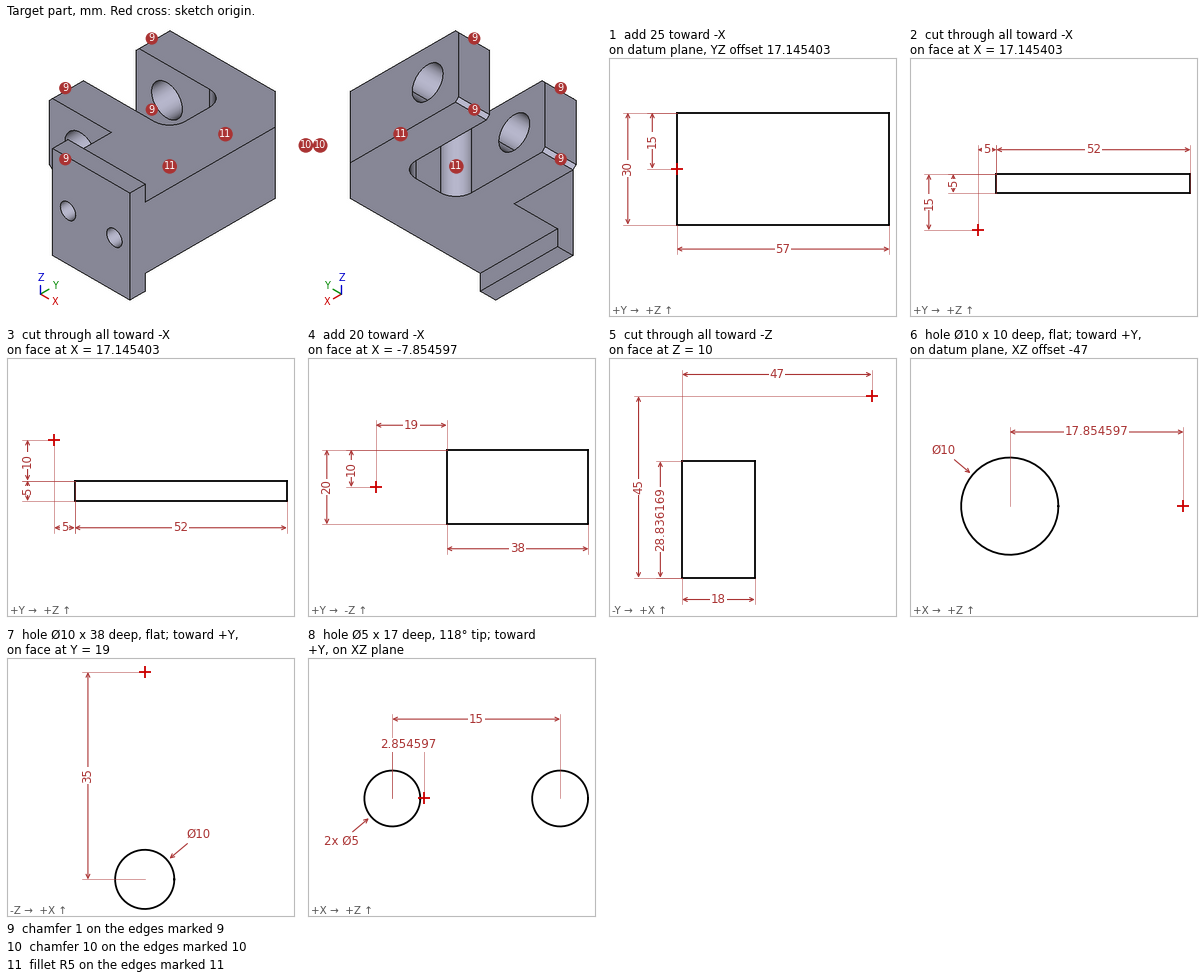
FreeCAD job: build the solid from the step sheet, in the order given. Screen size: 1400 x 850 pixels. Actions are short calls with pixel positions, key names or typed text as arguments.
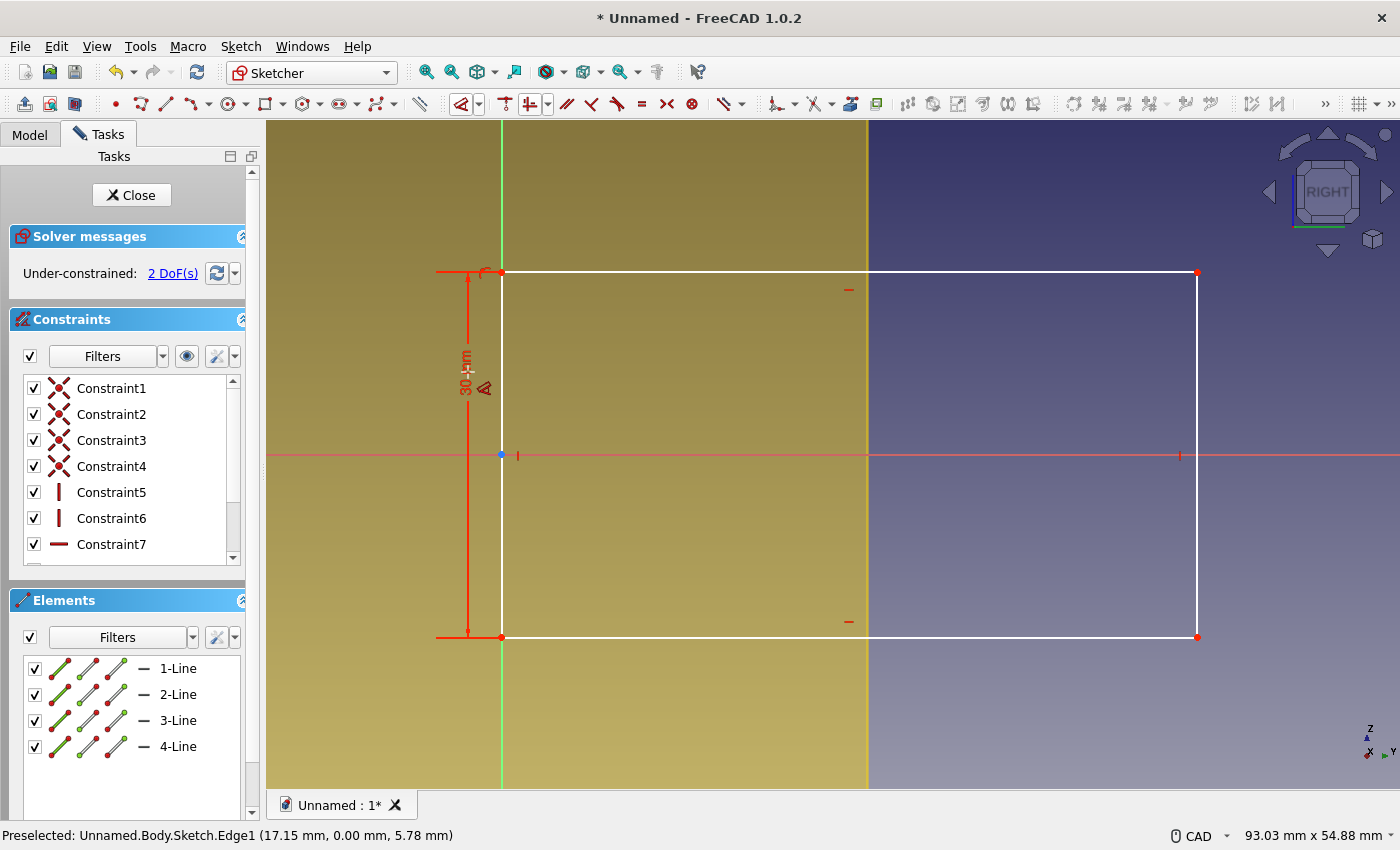
click(710, 638)
click(849, 672)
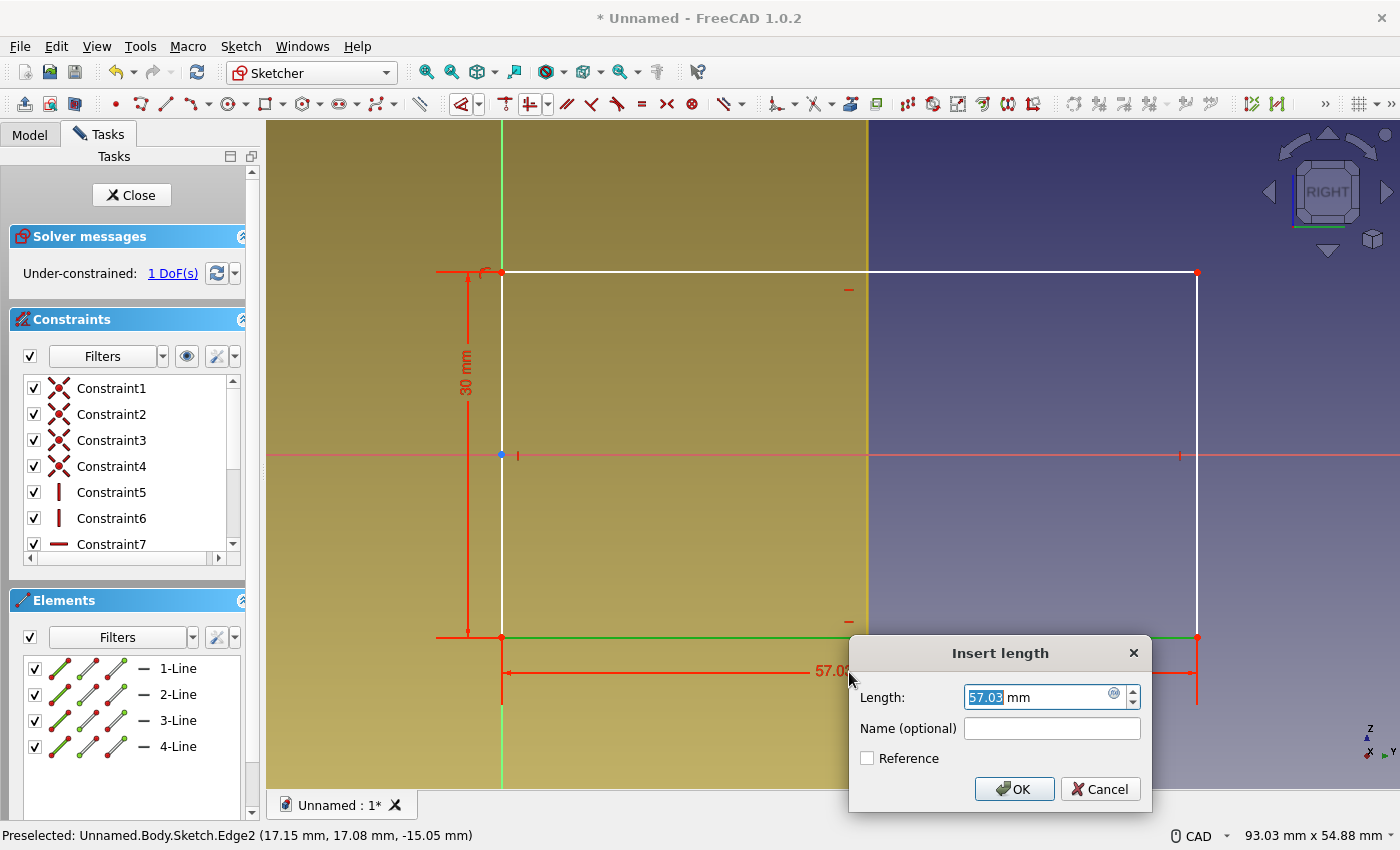
text(57)
key(Return)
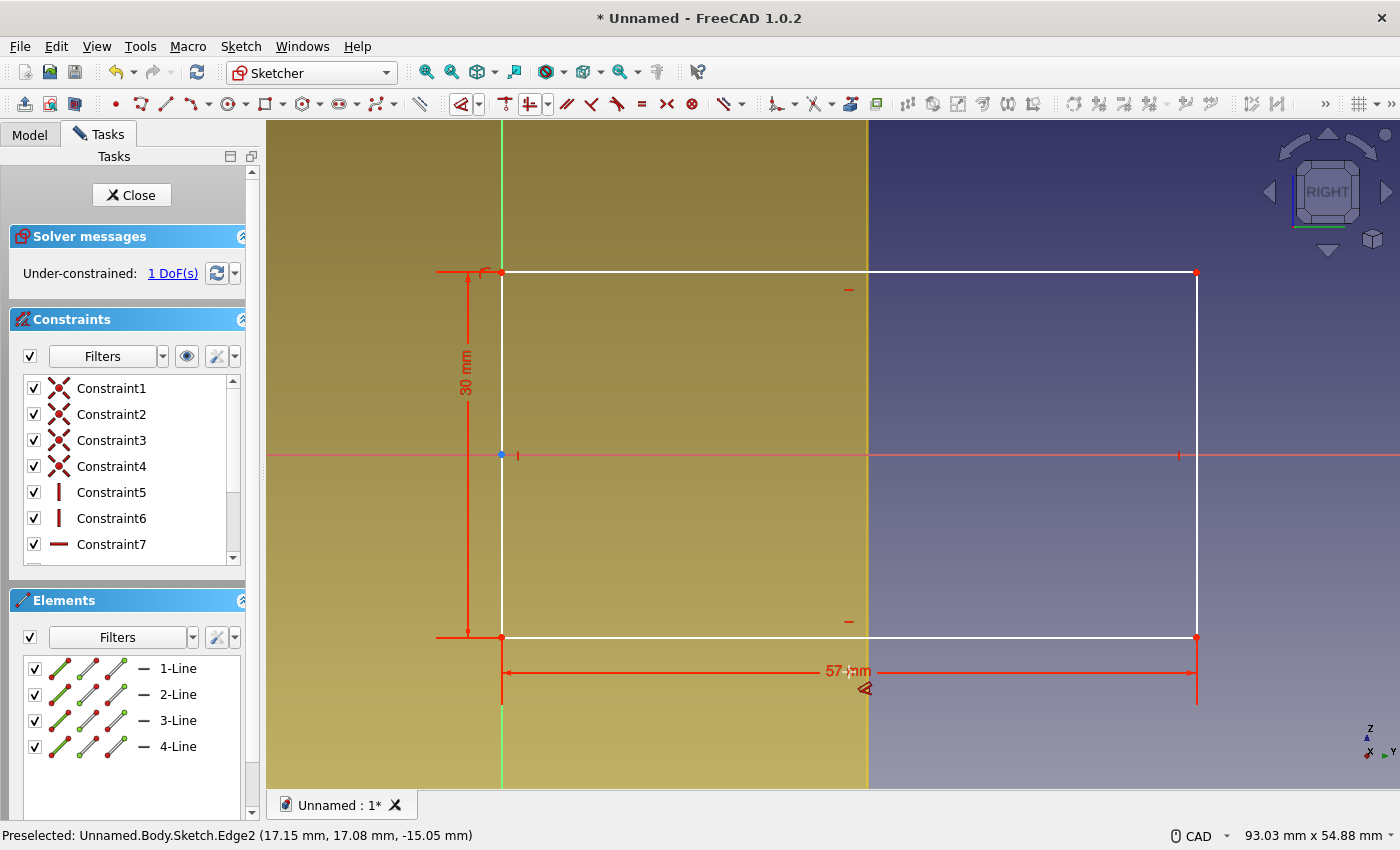
click(502, 272)
click(468, 321)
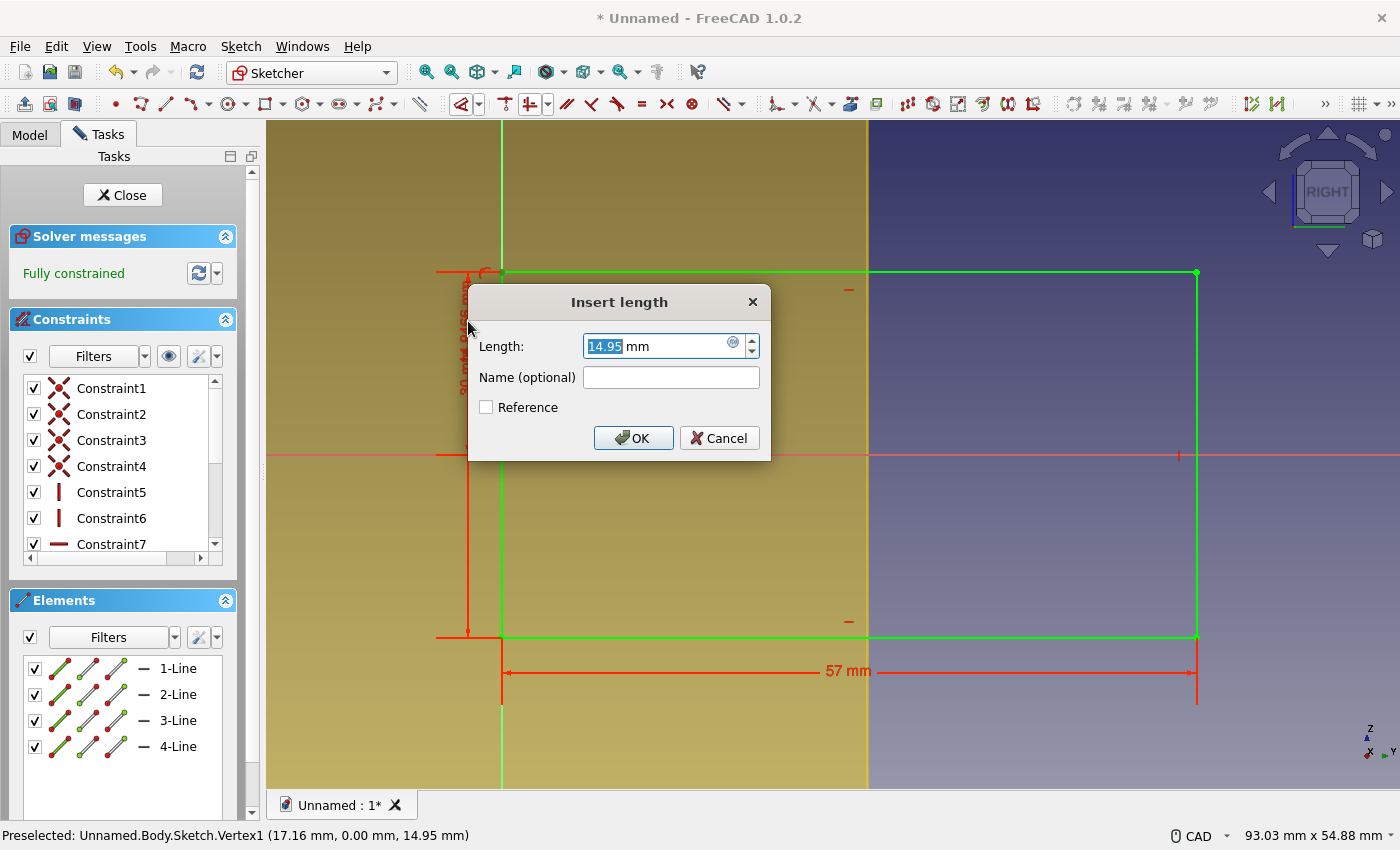
text(15)
key(Return)
key(Escape)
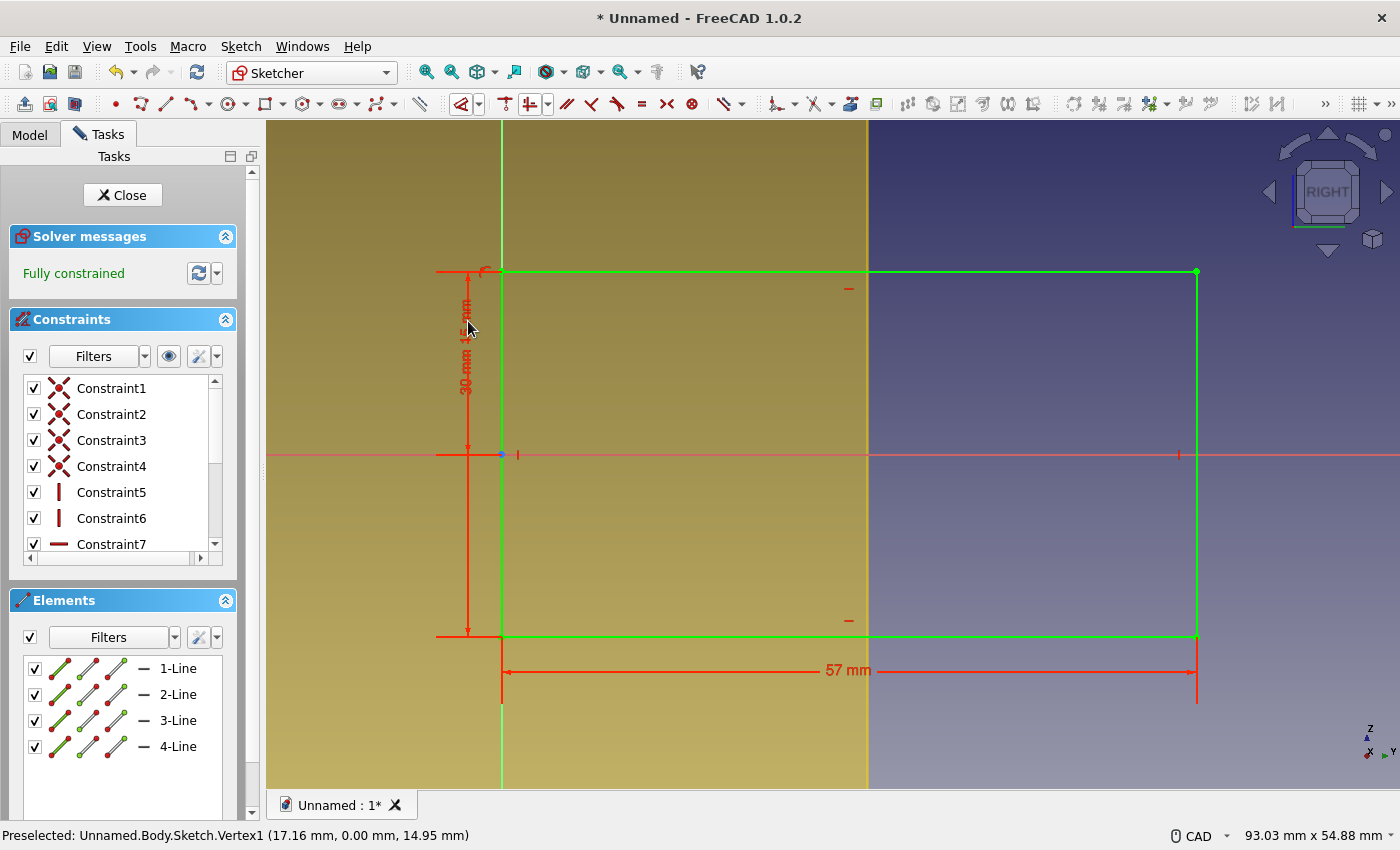
click(123, 195)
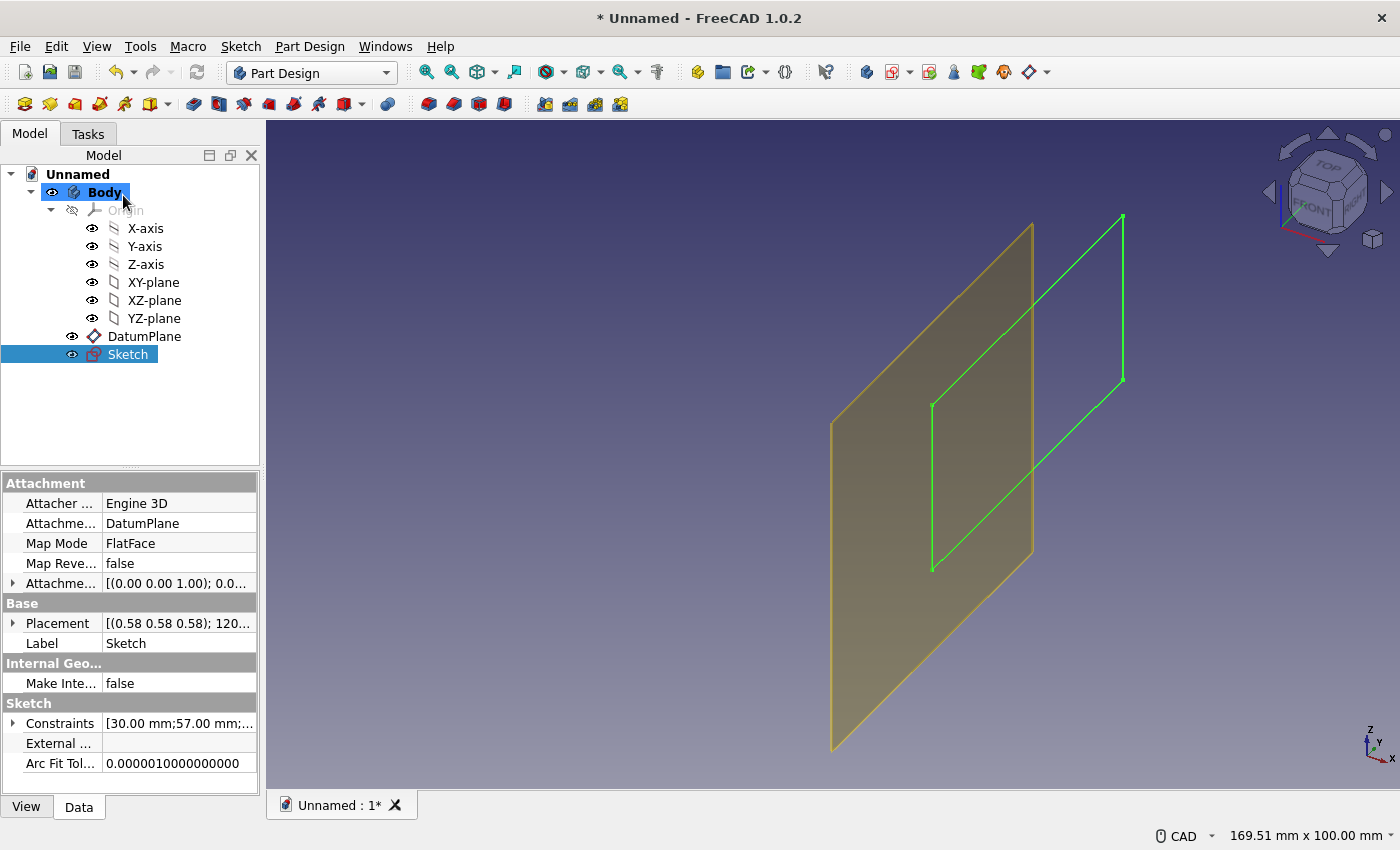
click(25, 104)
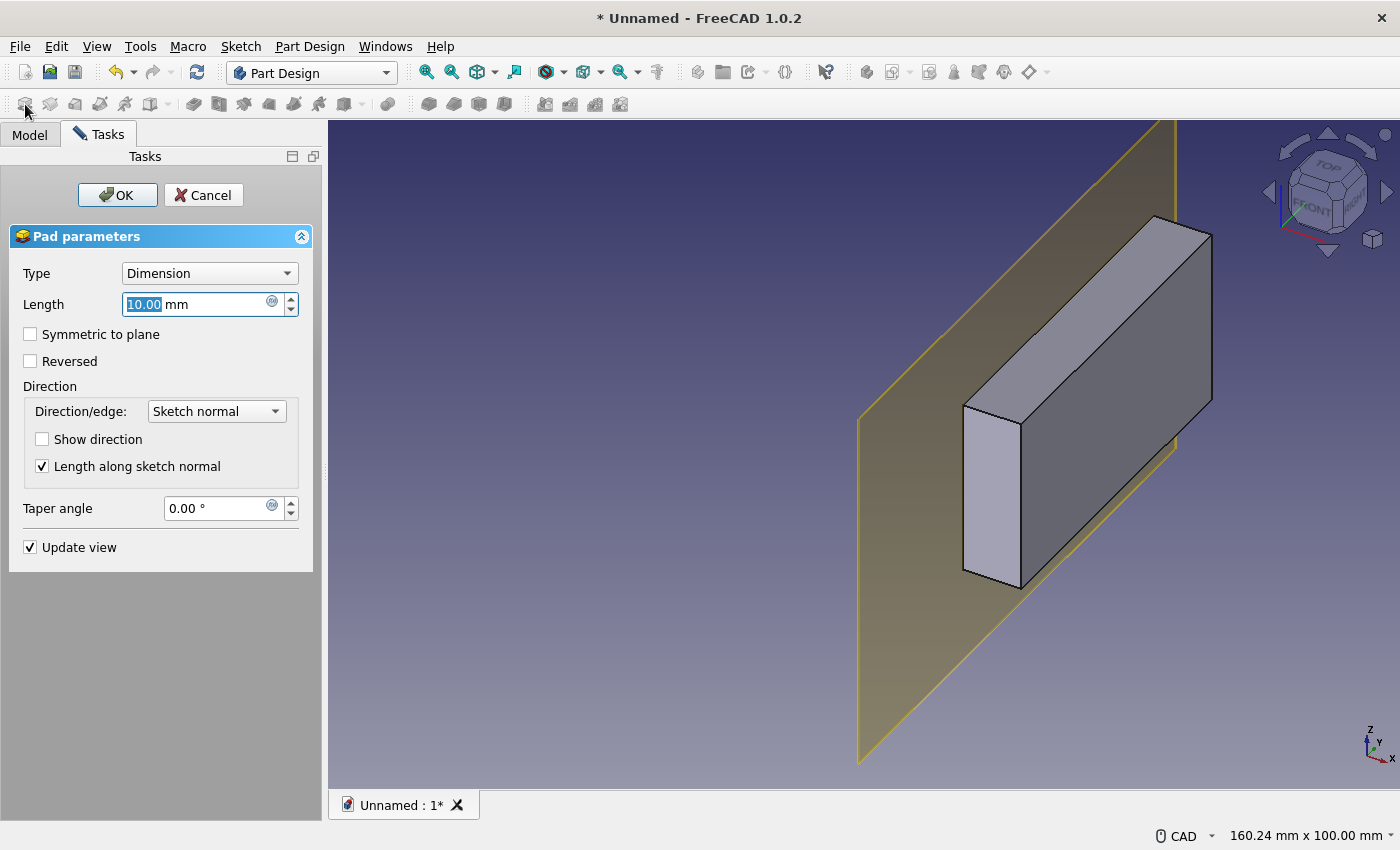
text(25)
key(Tab)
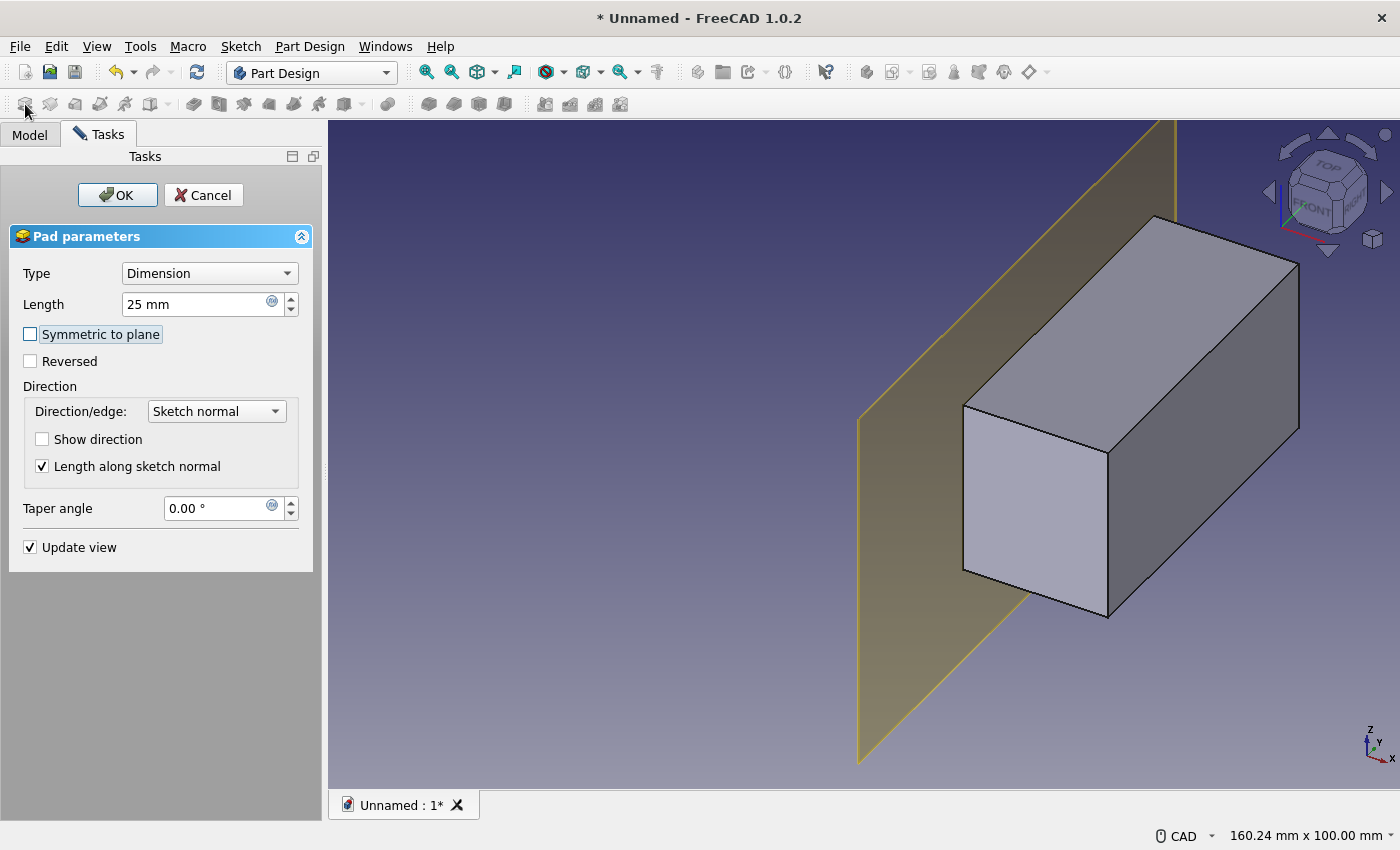
click(31, 361)